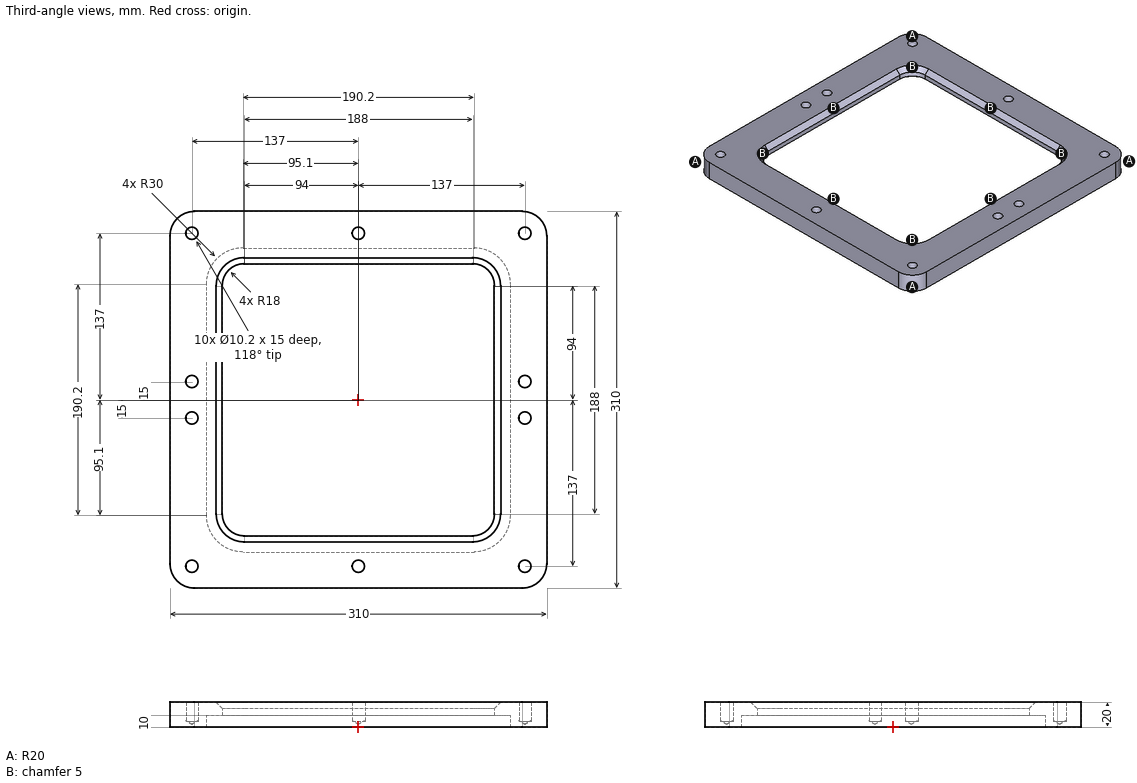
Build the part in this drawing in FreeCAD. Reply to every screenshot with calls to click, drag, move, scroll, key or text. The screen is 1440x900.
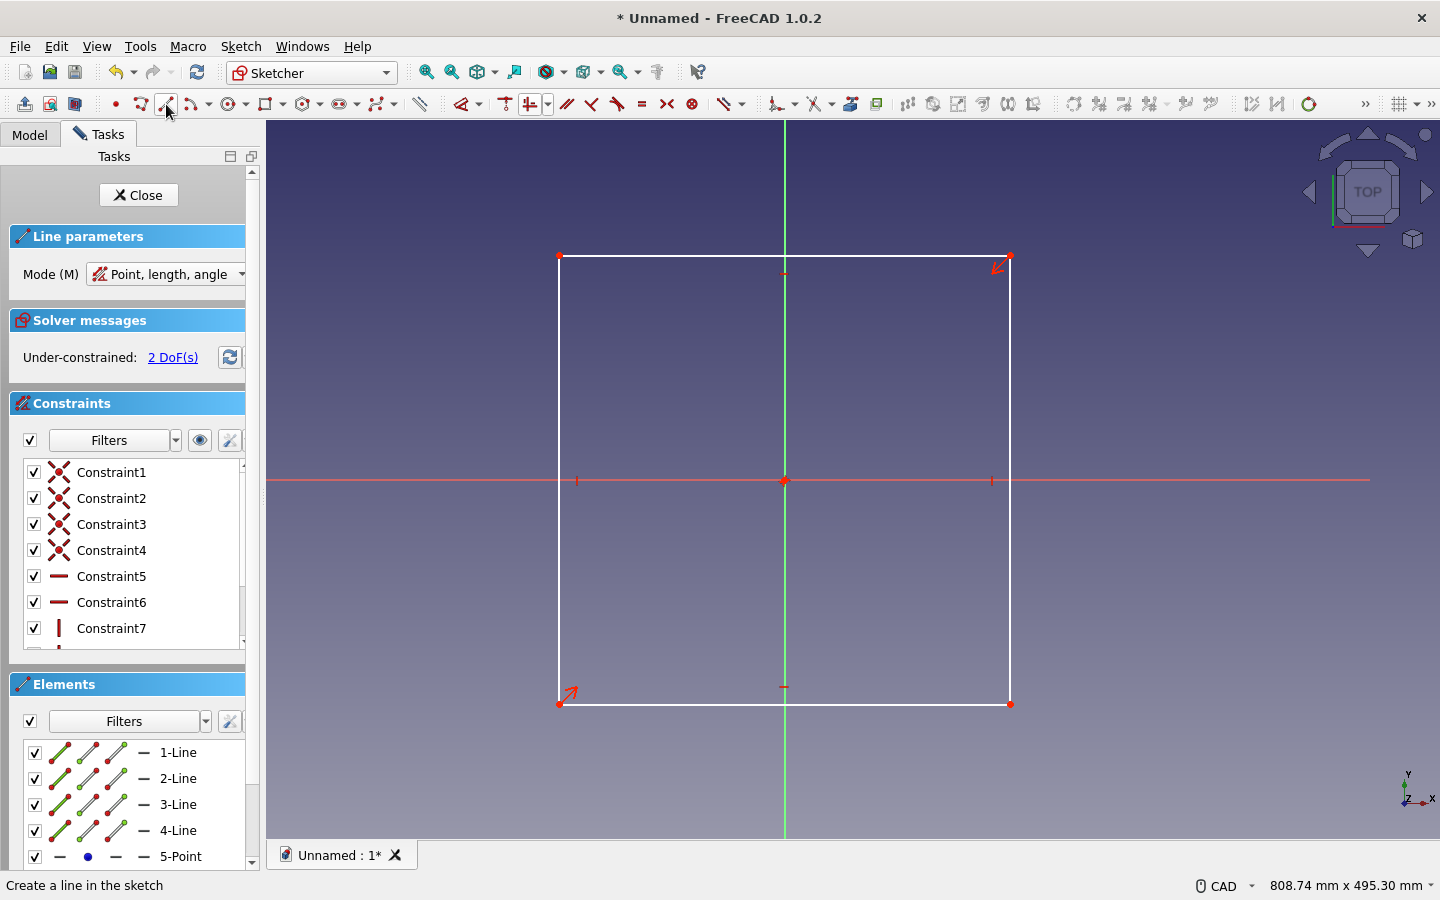
click(648, 318)
click(921, 318)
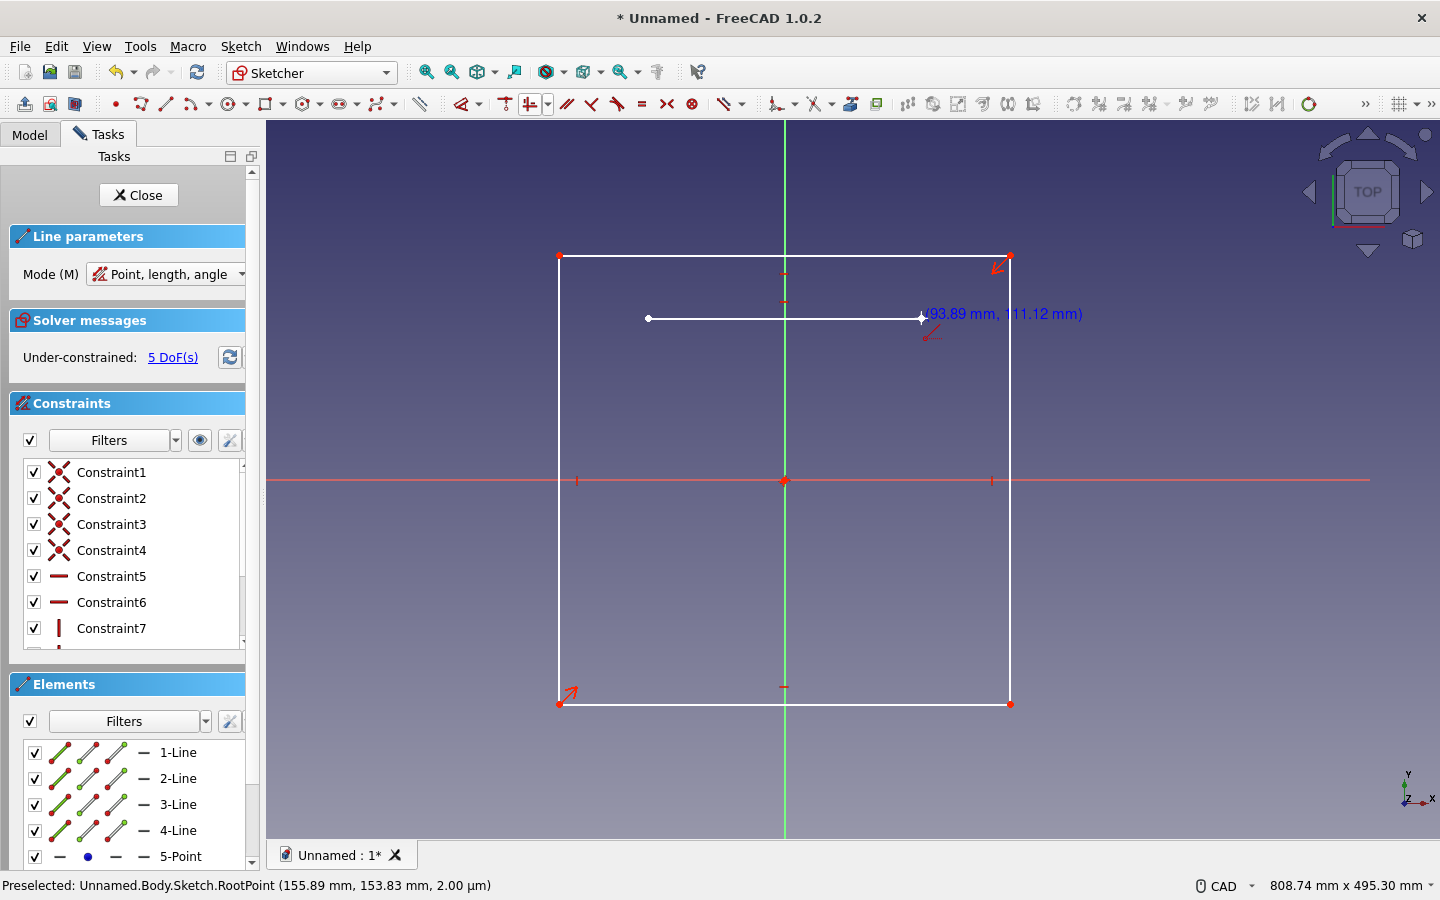
click(947, 344)
click(947, 617)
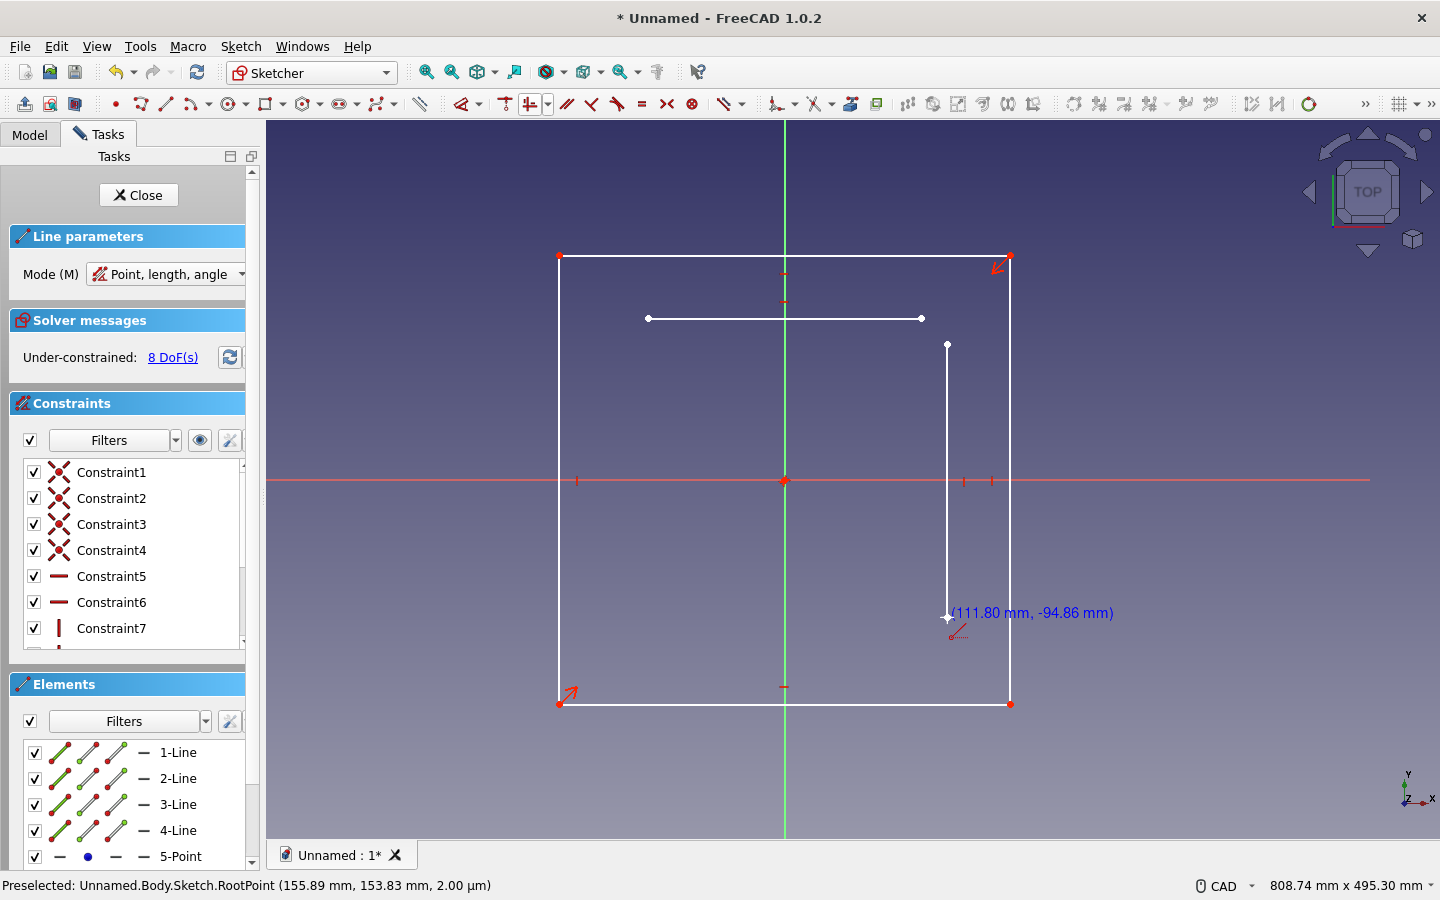
click(921, 643)
click(648, 643)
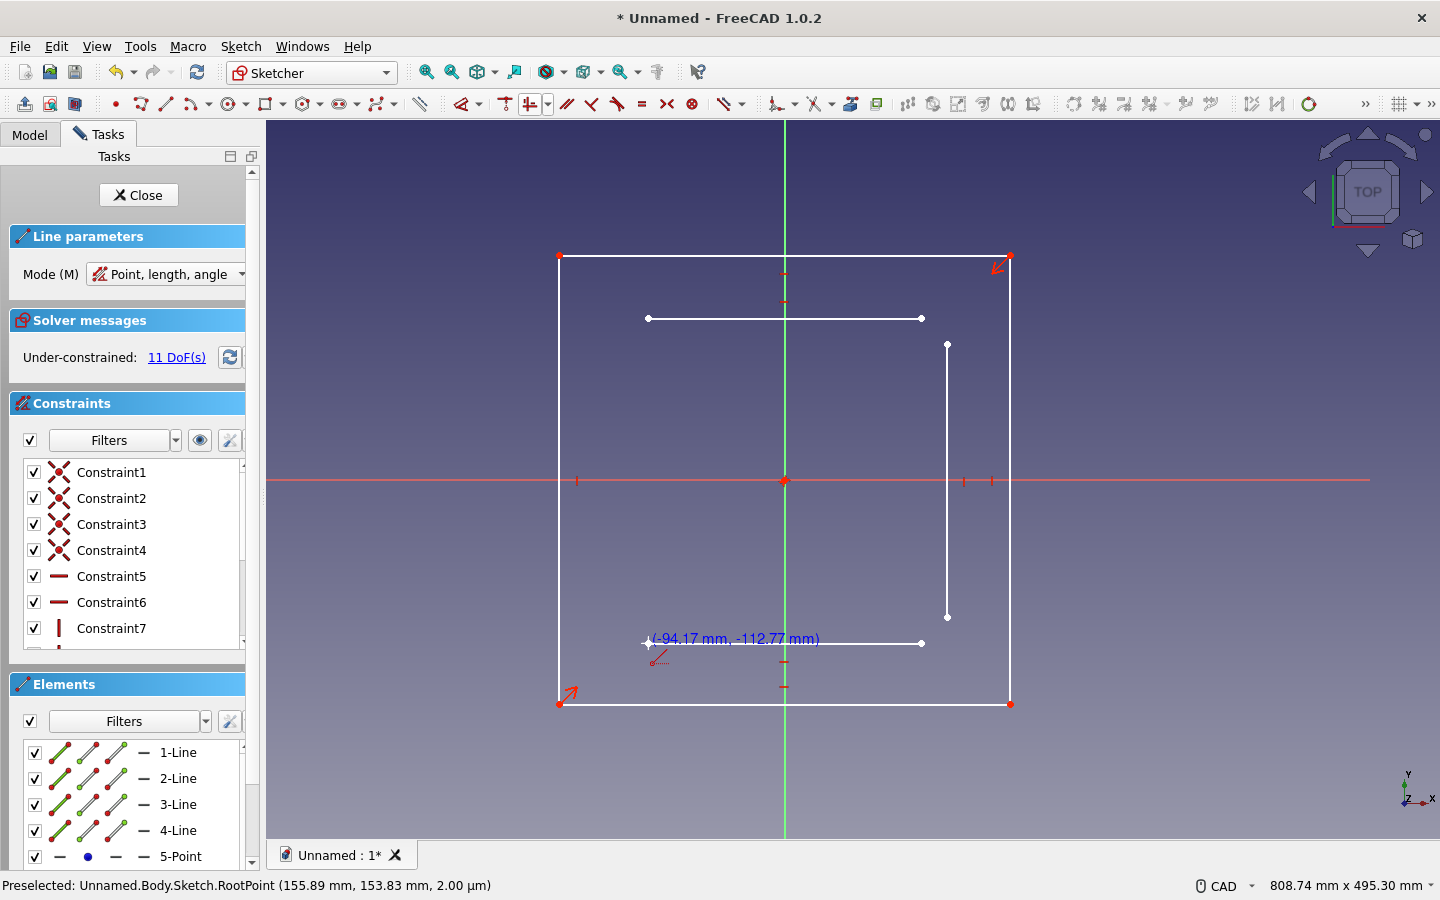
click(622, 617)
click(622, 344)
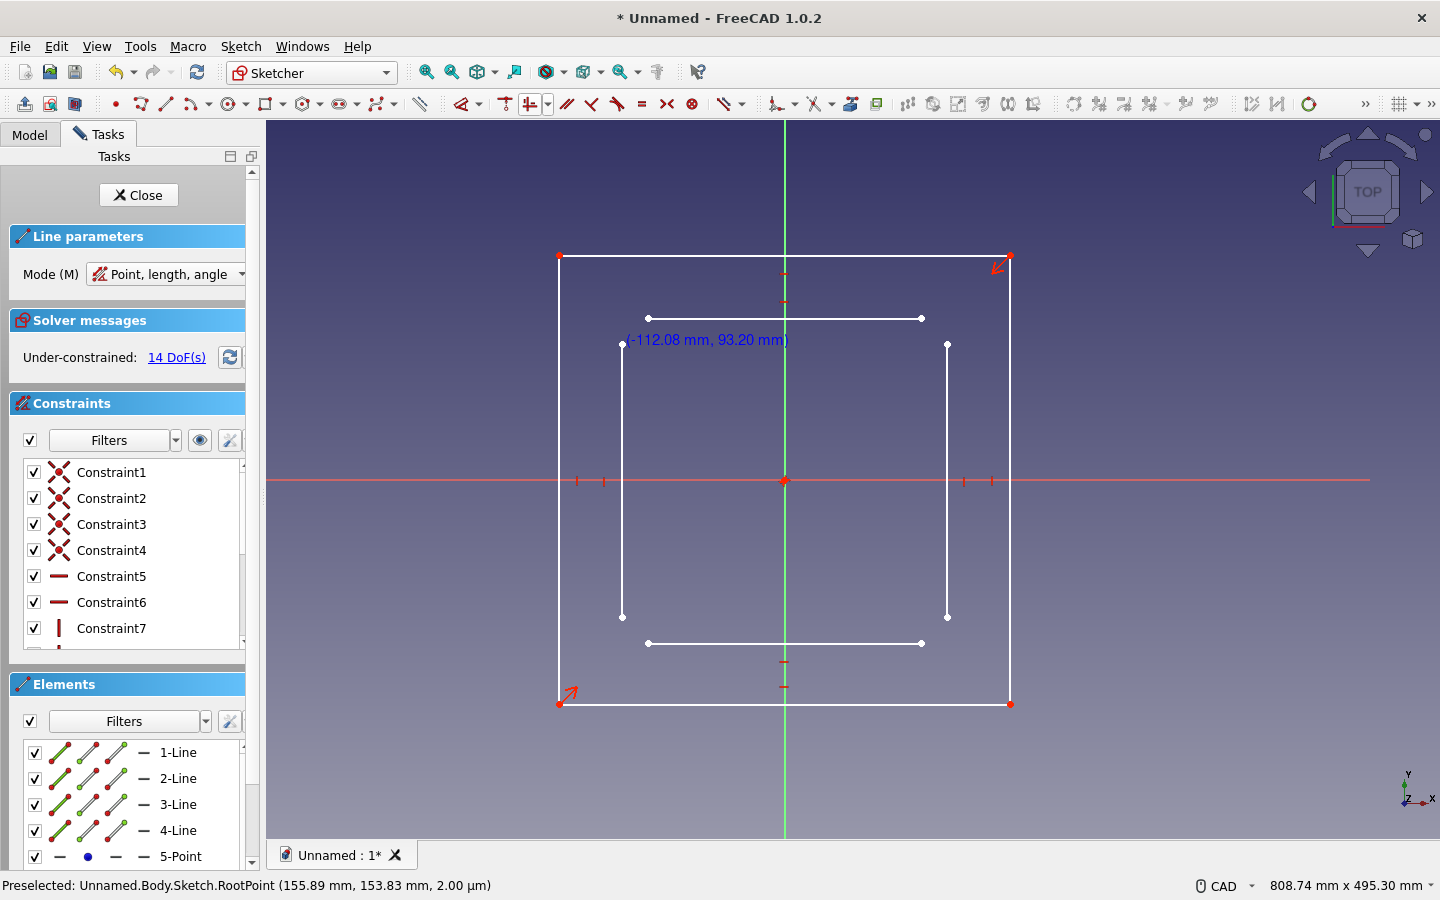
key(g)
key(3)
key(a)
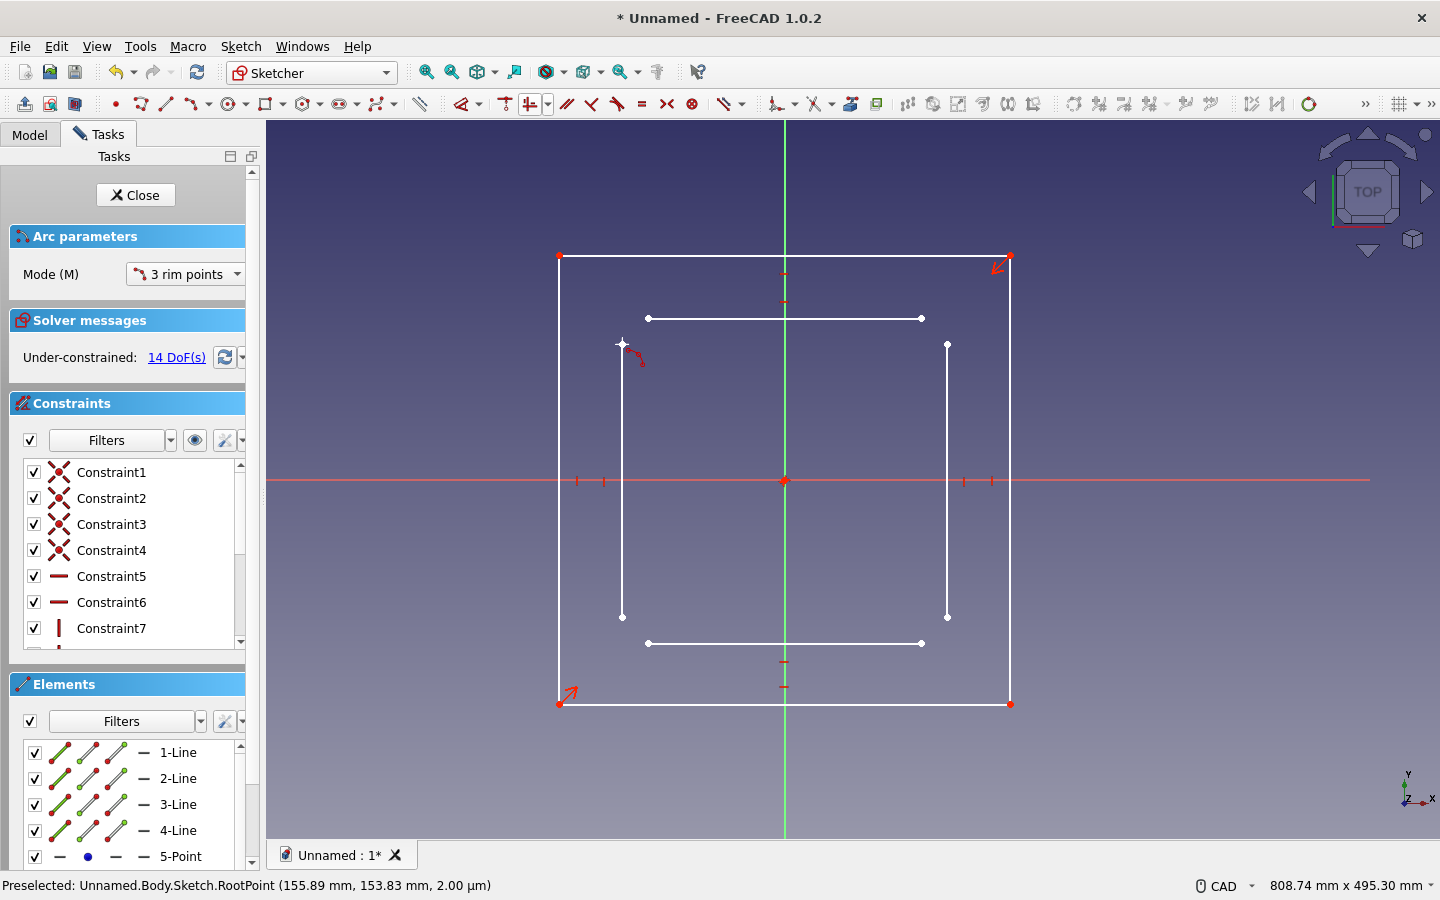
click(921, 319)
click(947, 345)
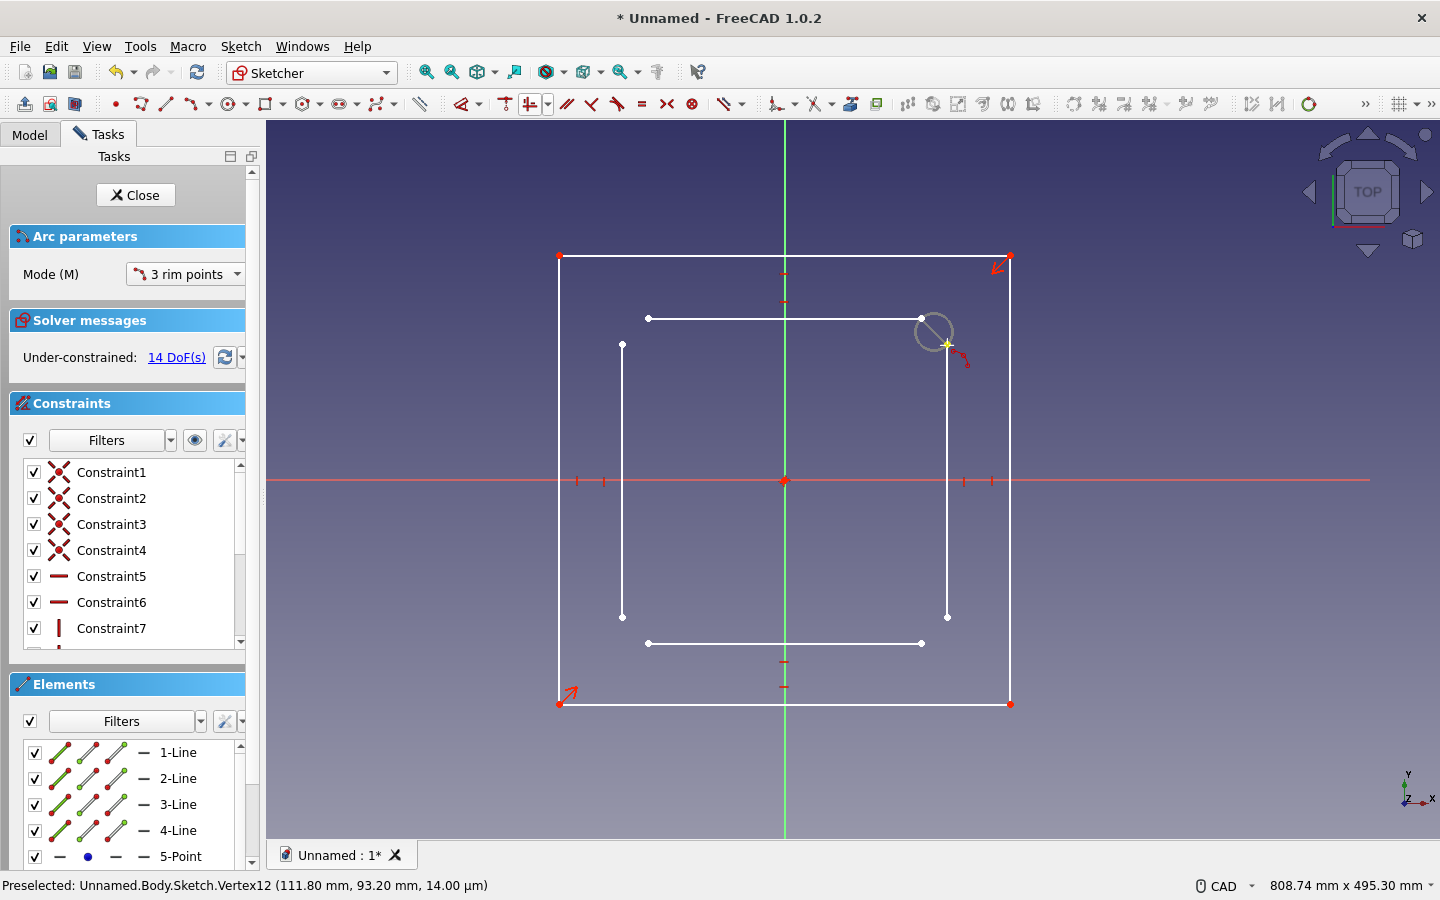
scroll(940, 325, up, 4)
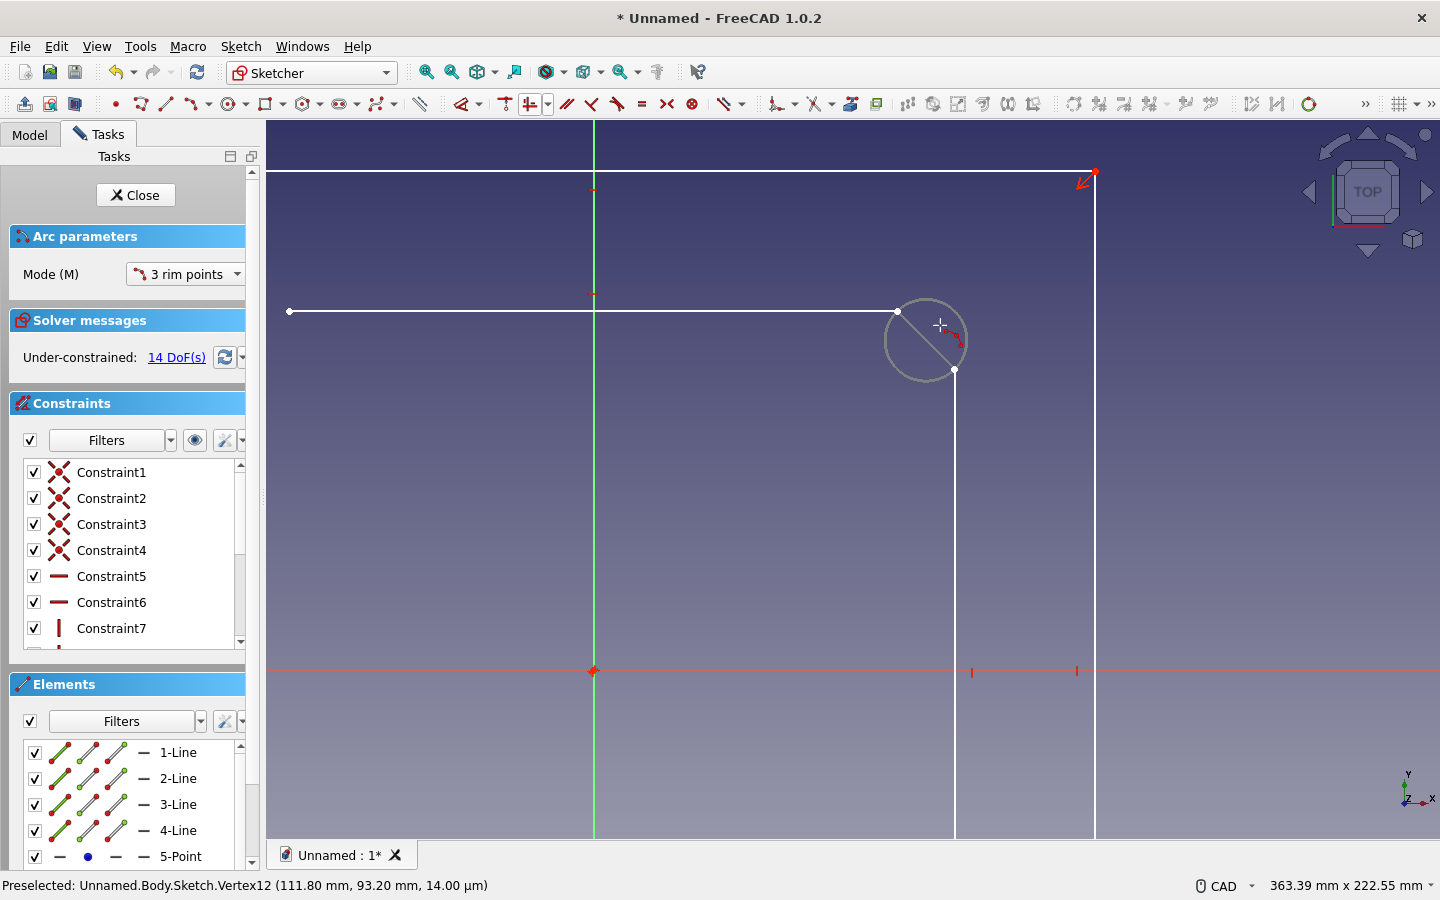
click(938, 325)